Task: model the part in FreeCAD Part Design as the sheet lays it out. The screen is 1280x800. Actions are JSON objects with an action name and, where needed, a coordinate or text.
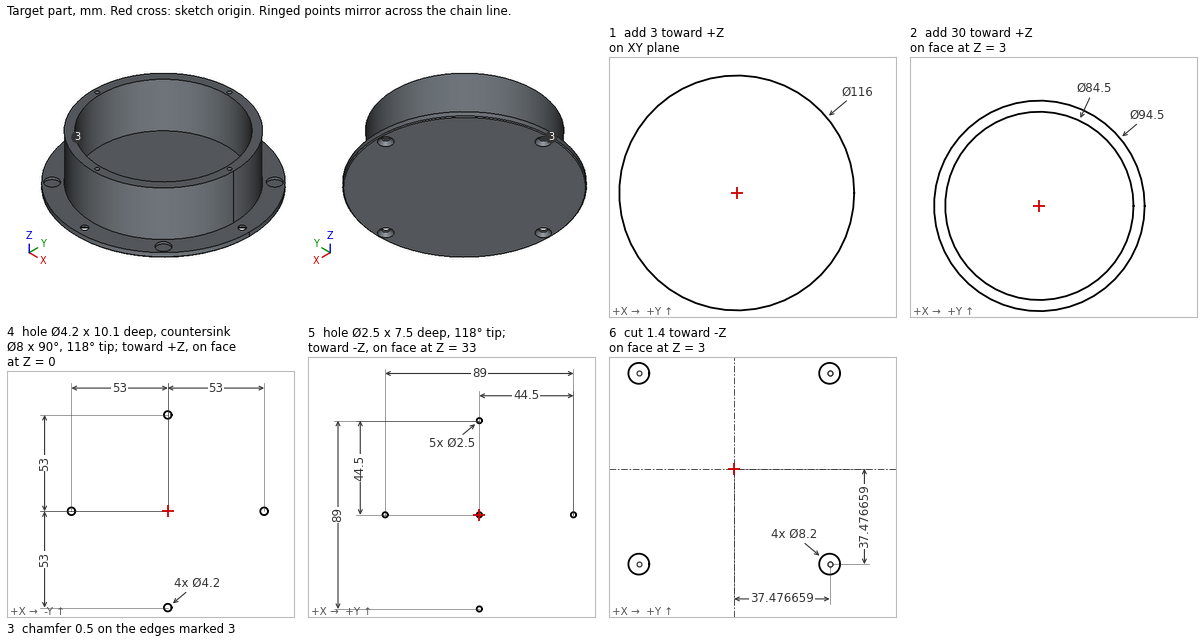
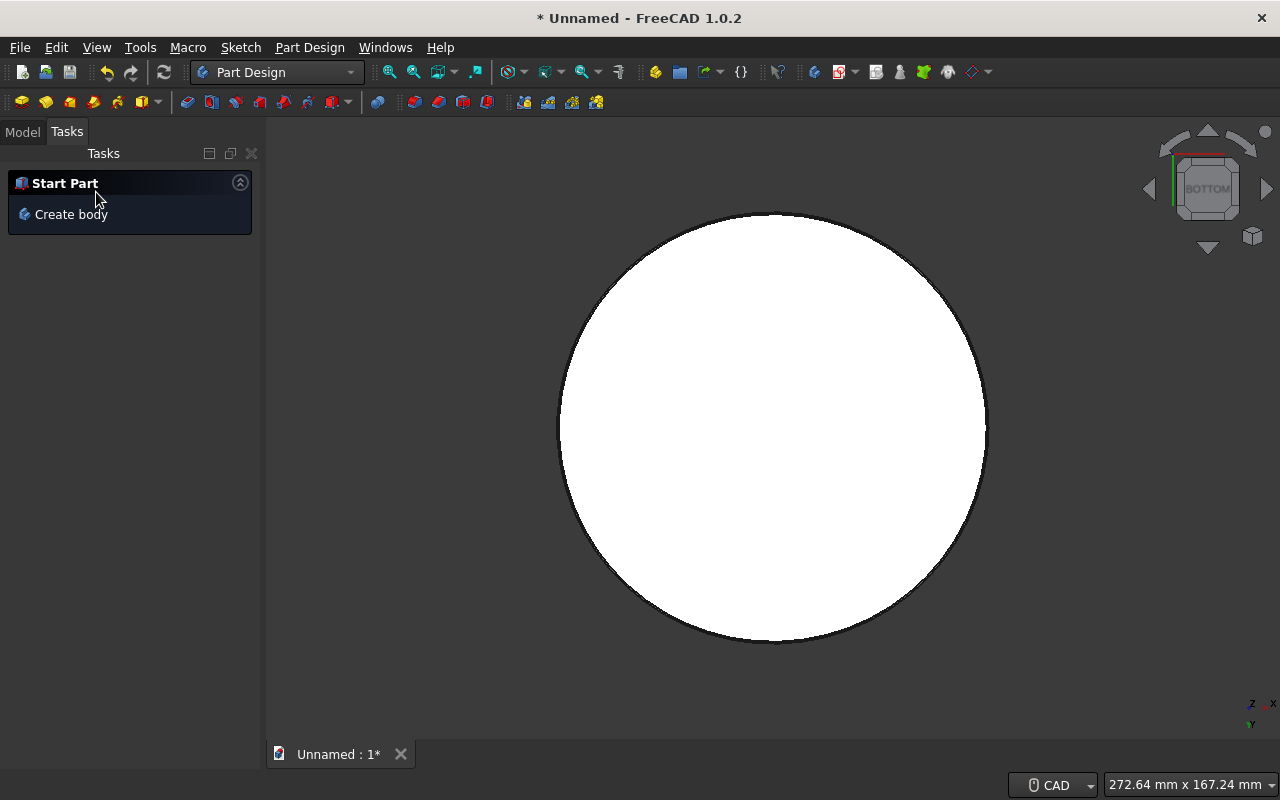
{"action": "left_click", "coordinate": [773, 427]}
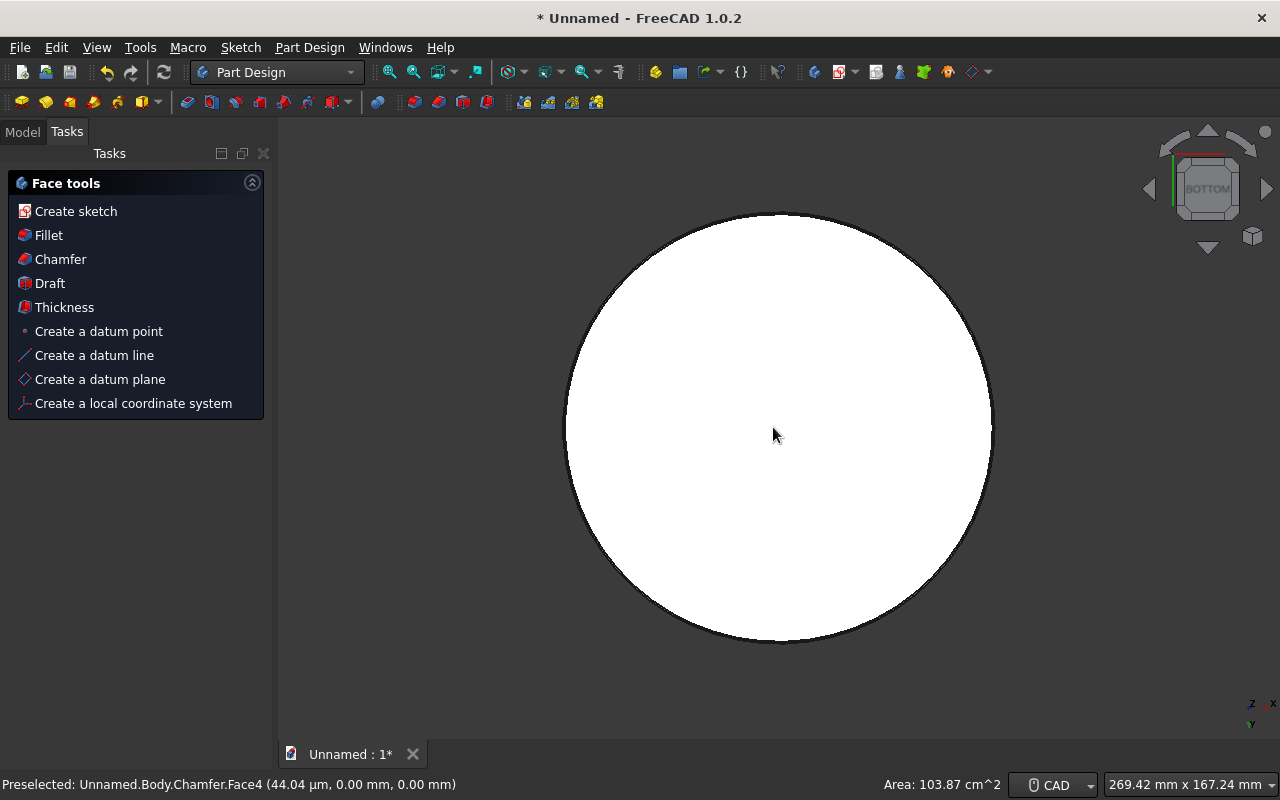
{"action": "left_click", "coordinate": [840, 72]}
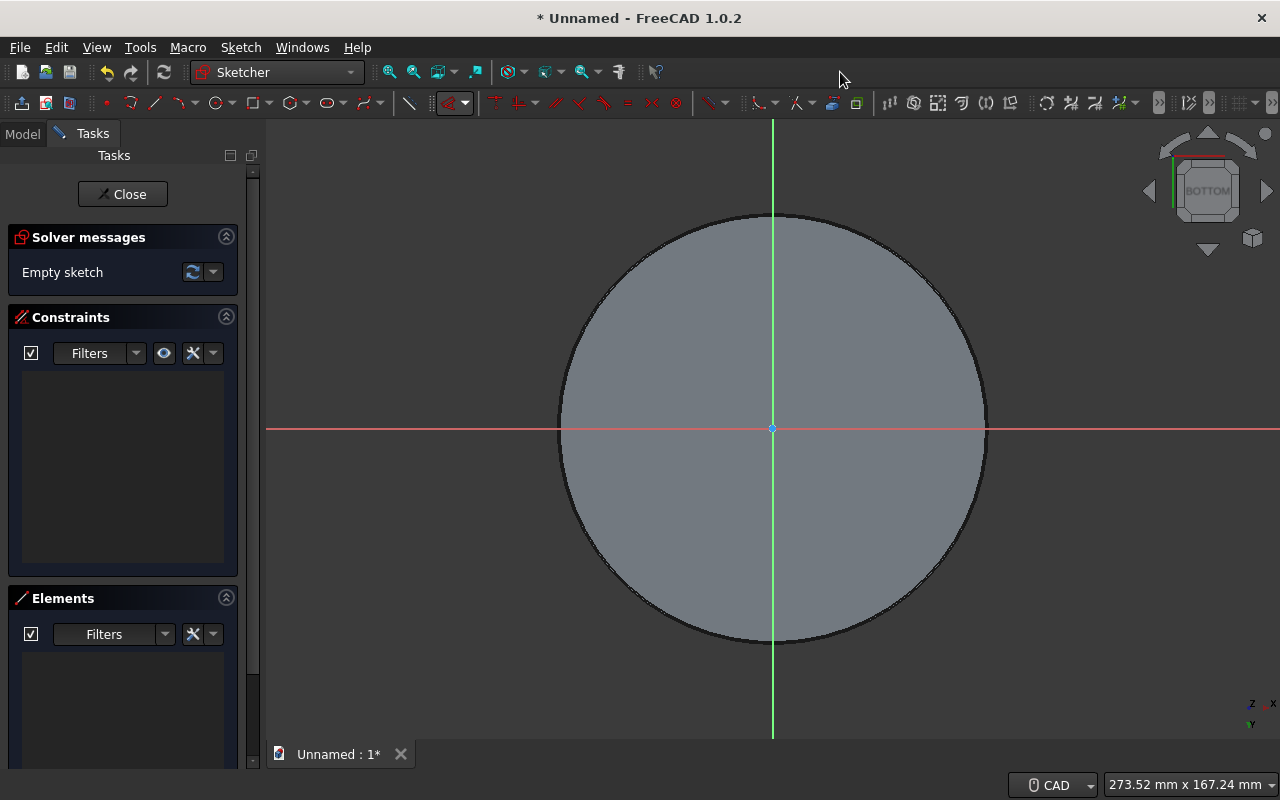
{"action": "left_click", "coordinate": [216, 104]}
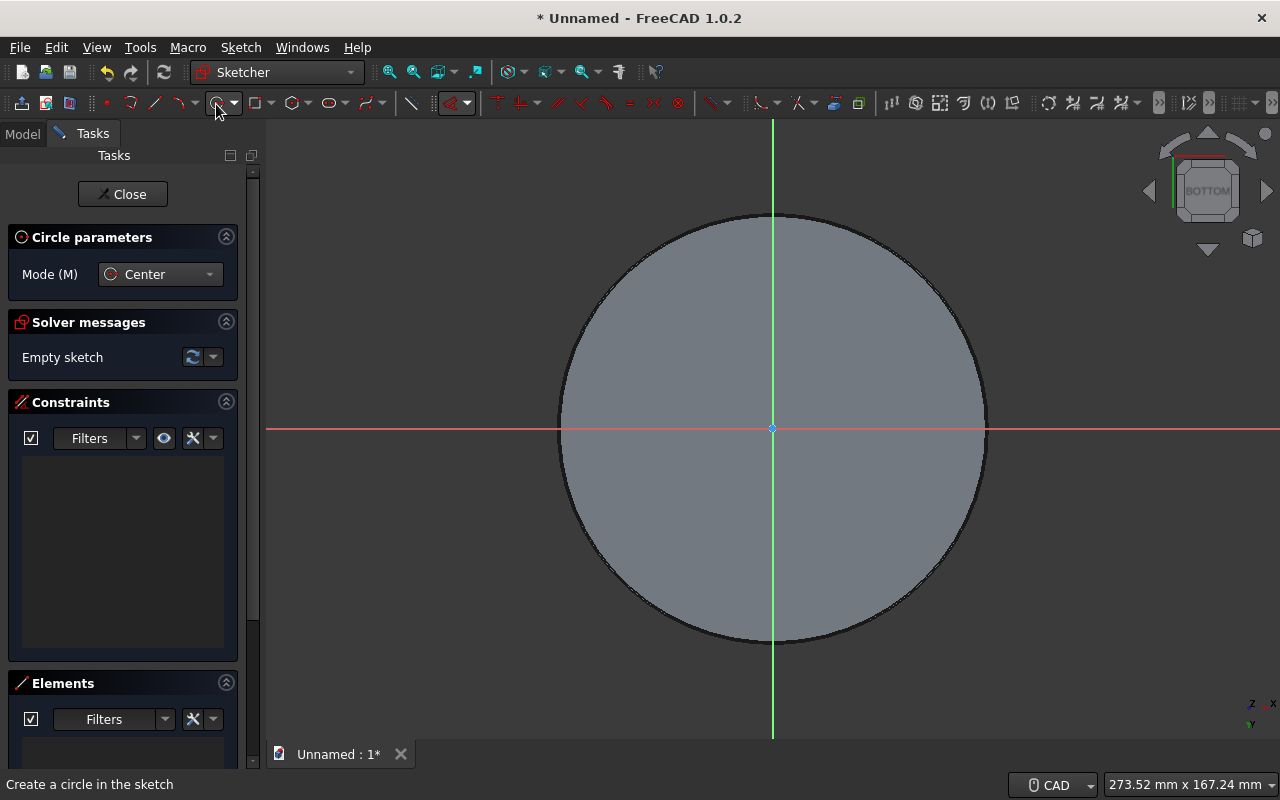
{"action": "scroll", "coordinate": [773, 625], "scroll_direction": "up", "scroll_amount": 6}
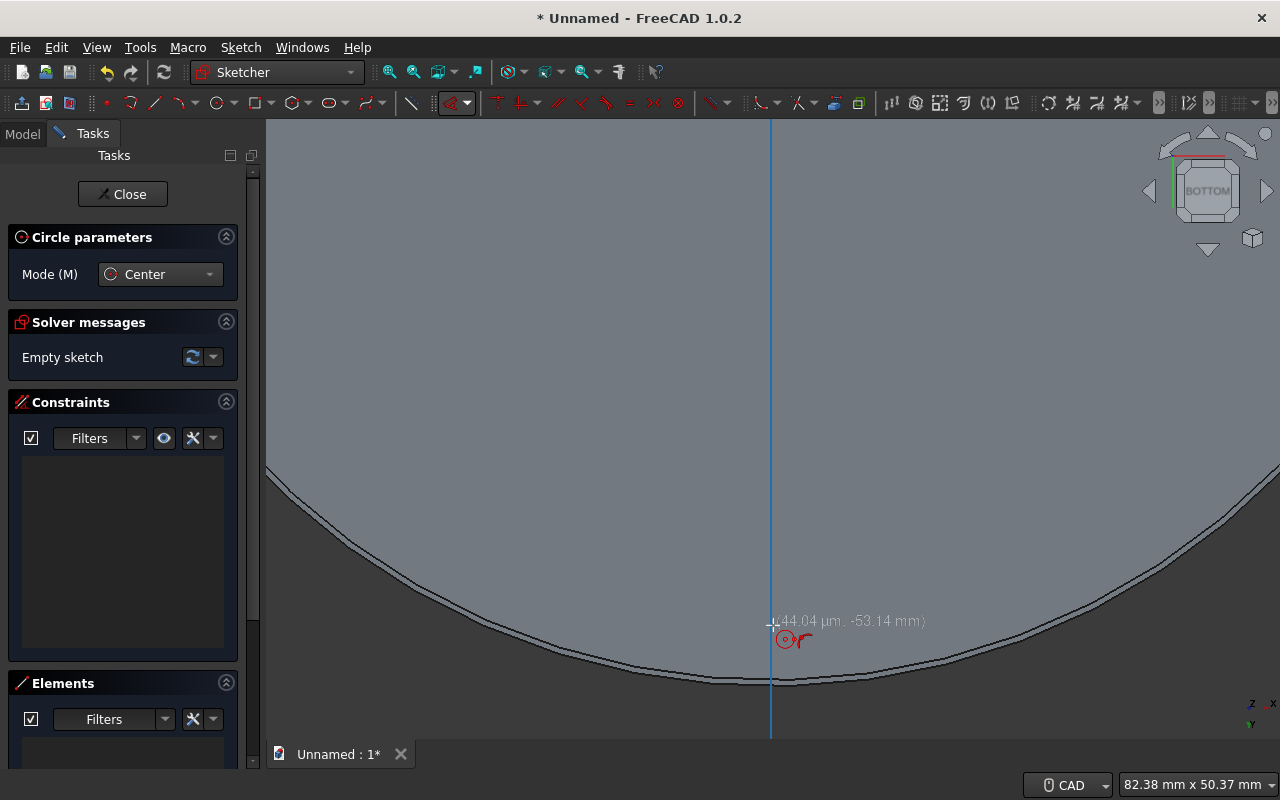
{"action": "left_click", "coordinate": [771, 625]}
{"action": "mouse_move", "coordinate": [790, 606]}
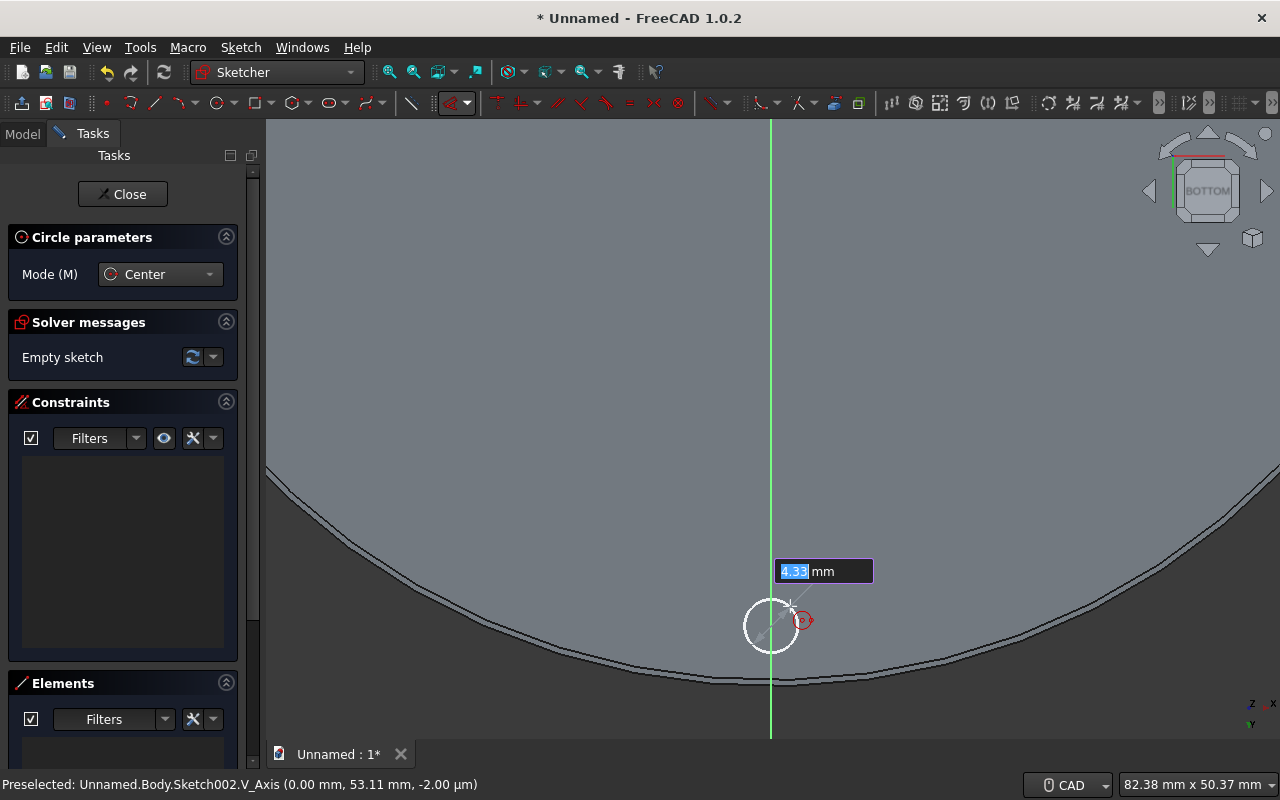
{"action": "type", "text": "4.2"}
{"action": "key", "text": "Return"}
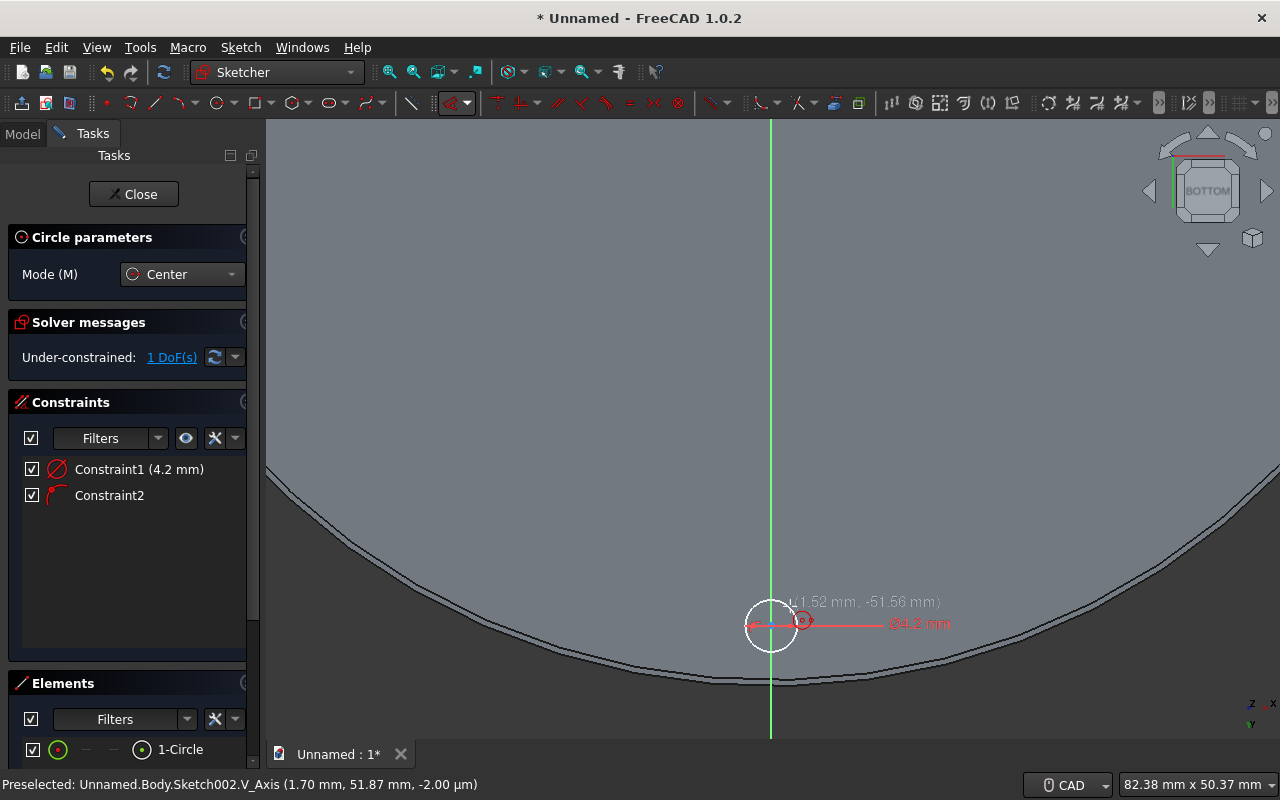
{"action": "scroll", "coordinate": [676, 626], "scroll_direction": "down", "scroll_amount": 6}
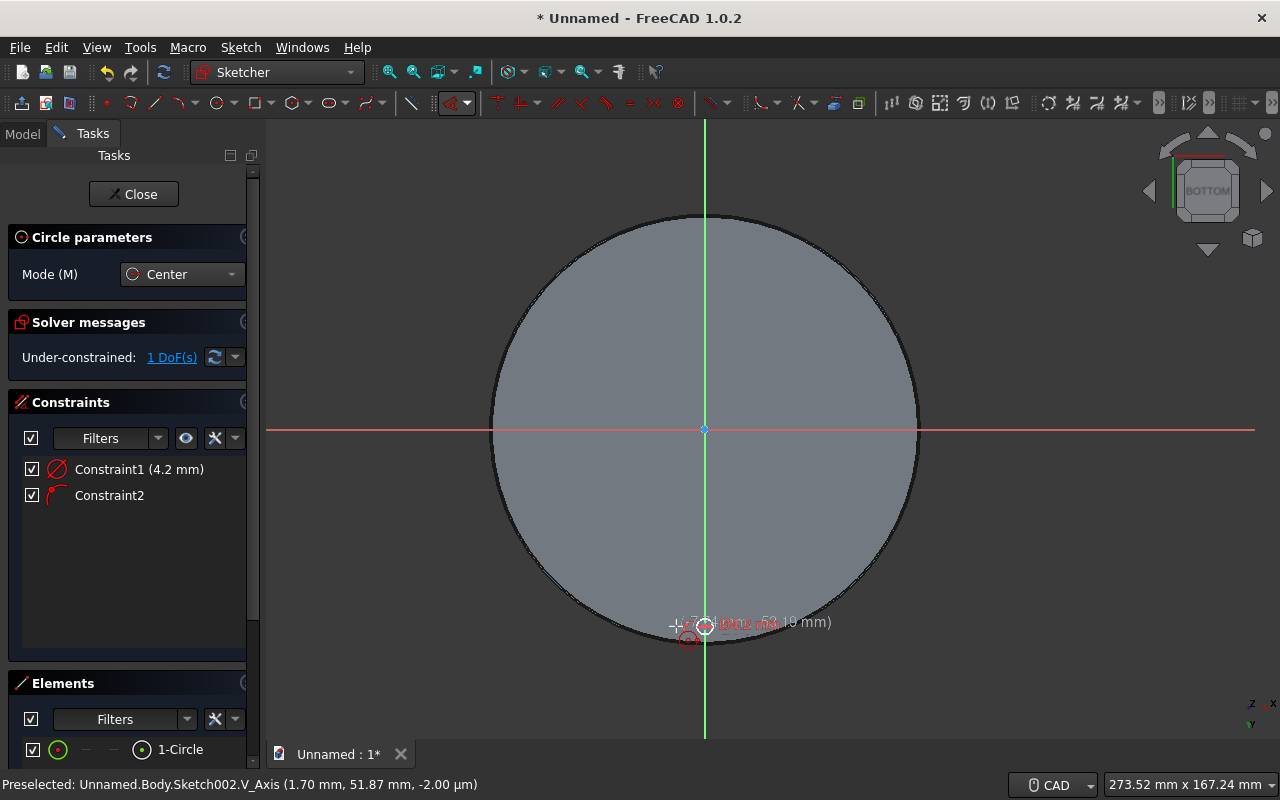
{"action": "scroll", "coordinate": [509, 430], "scroll_direction": "up", "scroll_amount": 6}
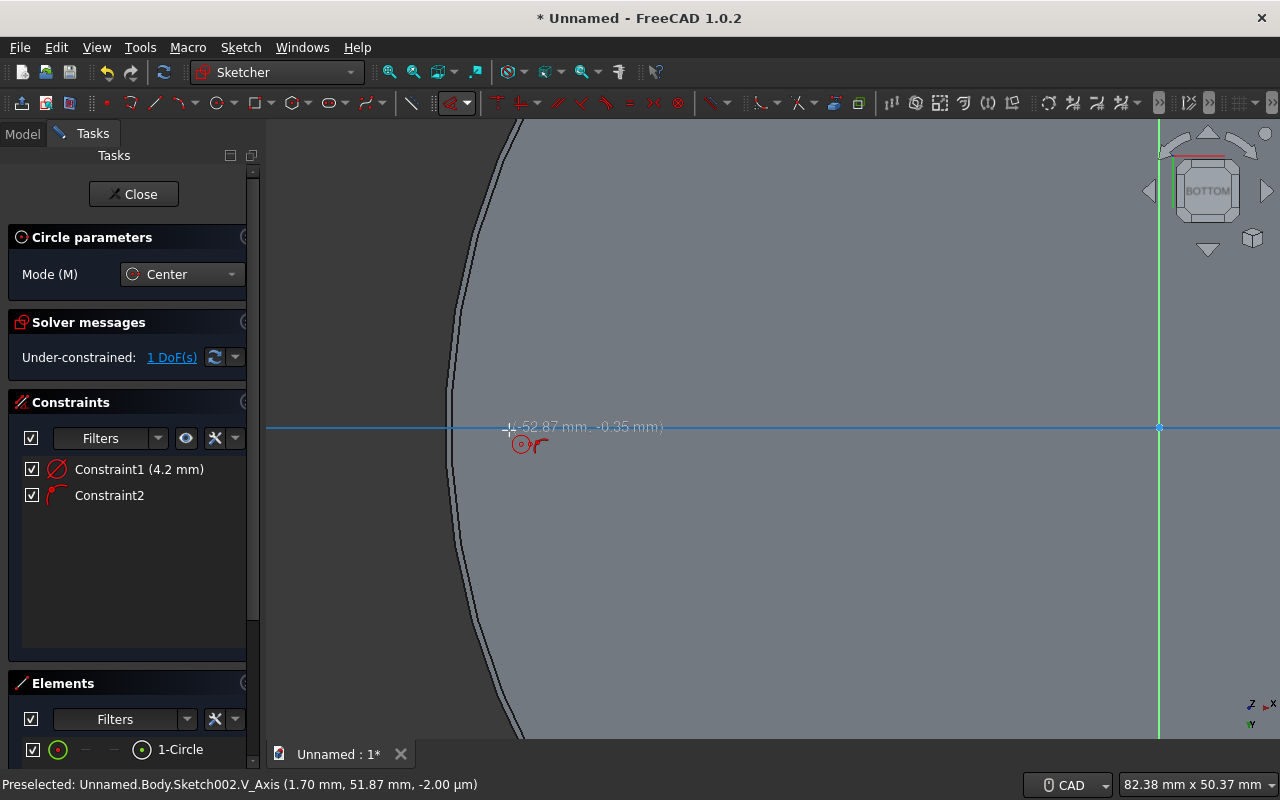
{"action": "left_click", "coordinate": [507, 428]}
{"action": "mouse_move", "coordinate": [525, 410]}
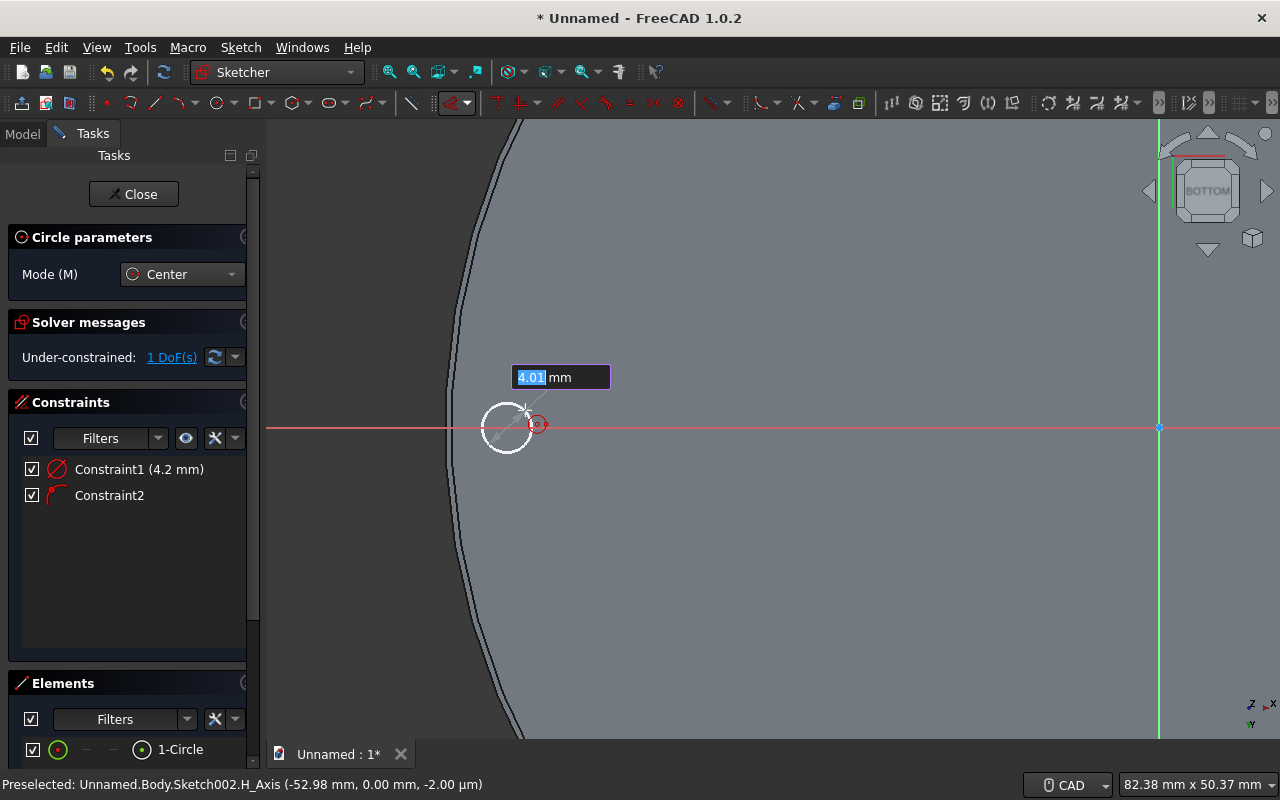
{"action": "type", "text": "4.2"}
{"action": "key", "text": "Return"}